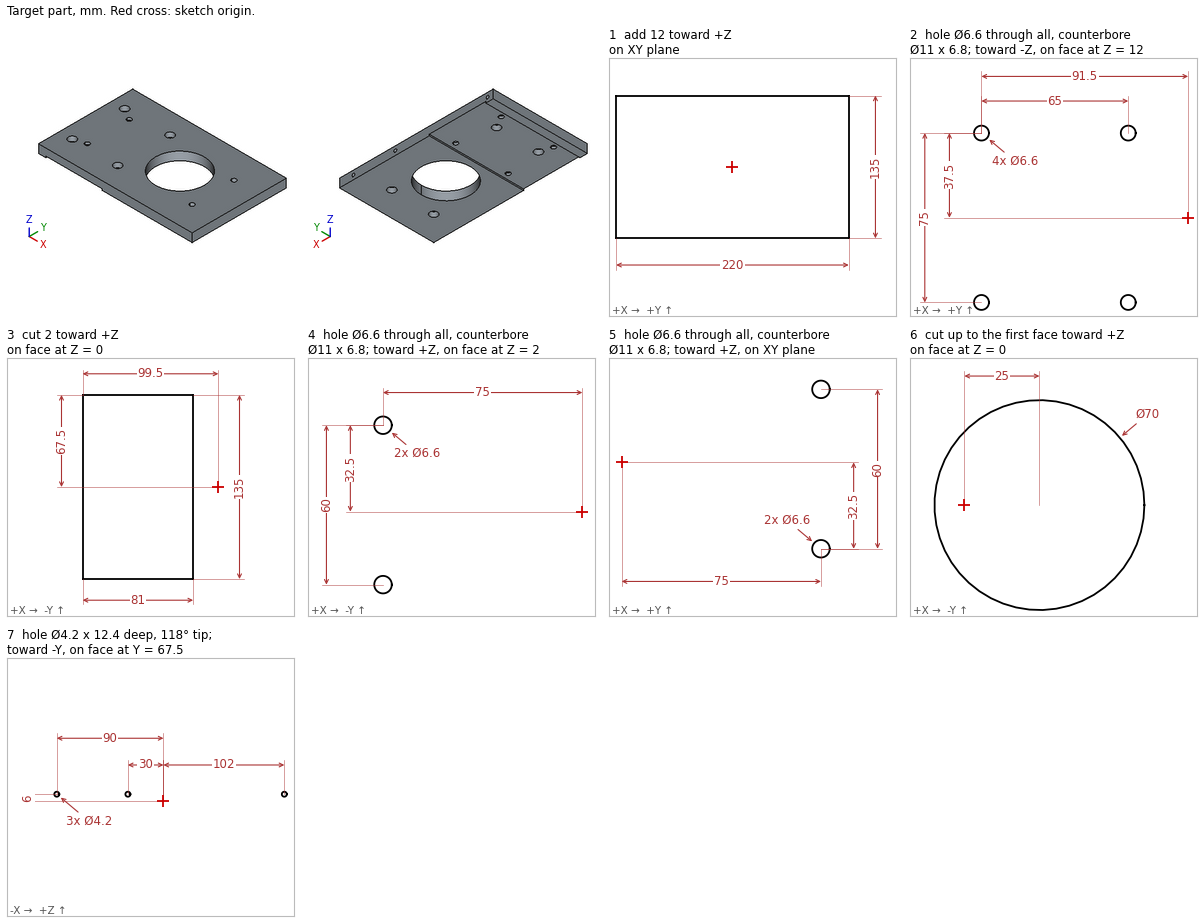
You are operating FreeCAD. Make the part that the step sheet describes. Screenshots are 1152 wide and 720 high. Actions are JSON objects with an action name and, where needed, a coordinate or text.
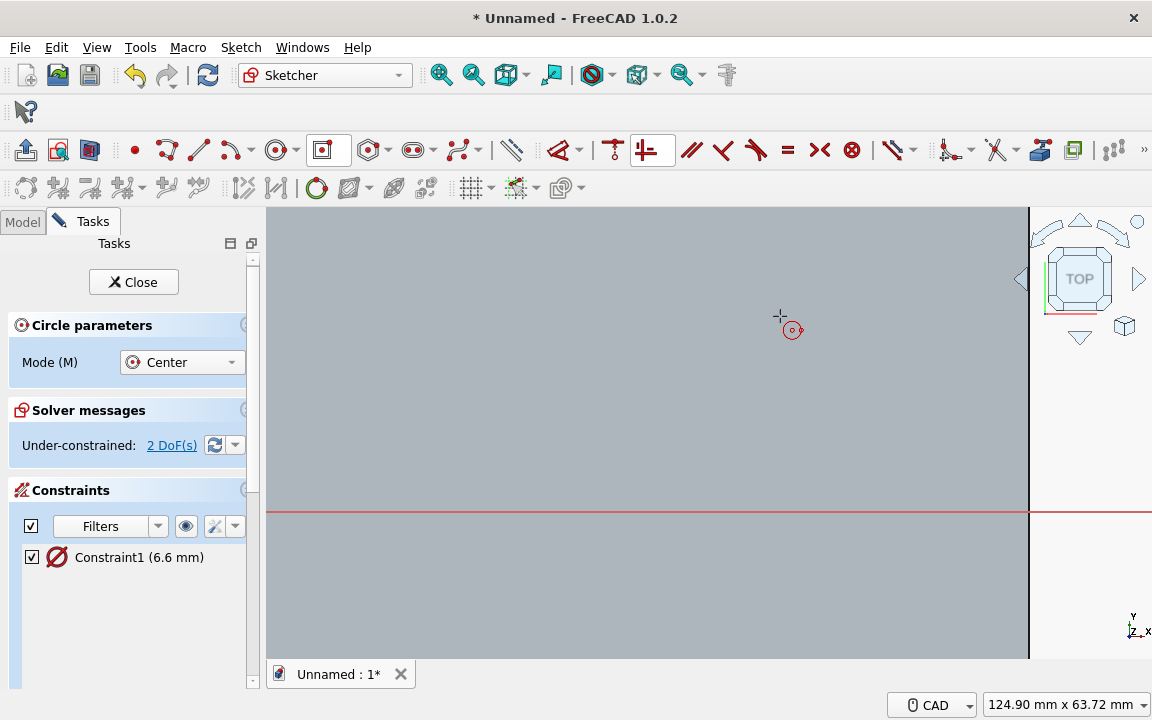
{"action": "left_click", "coordinate": [780, 317]}
{"action": "mouse_move", "coordinate": [797, 300]}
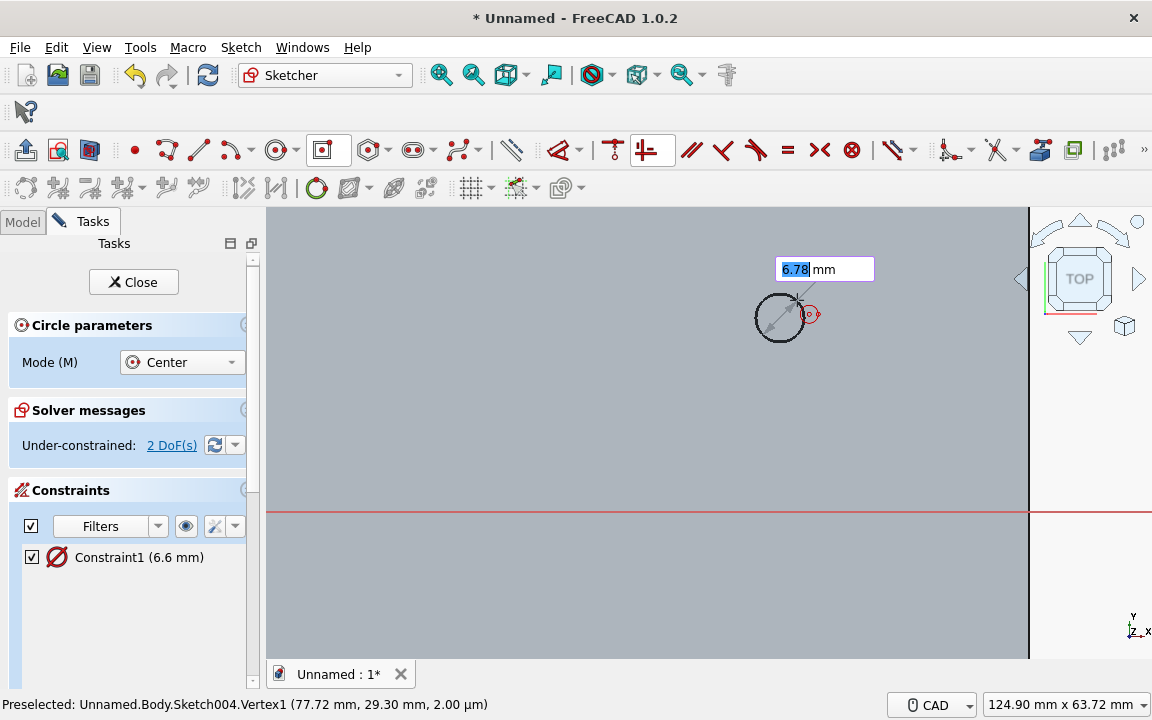
{"action": "type", "text": "6.6"}
{"action": "key", "text": "Return"}
{"action": "key", "text": "Escape"}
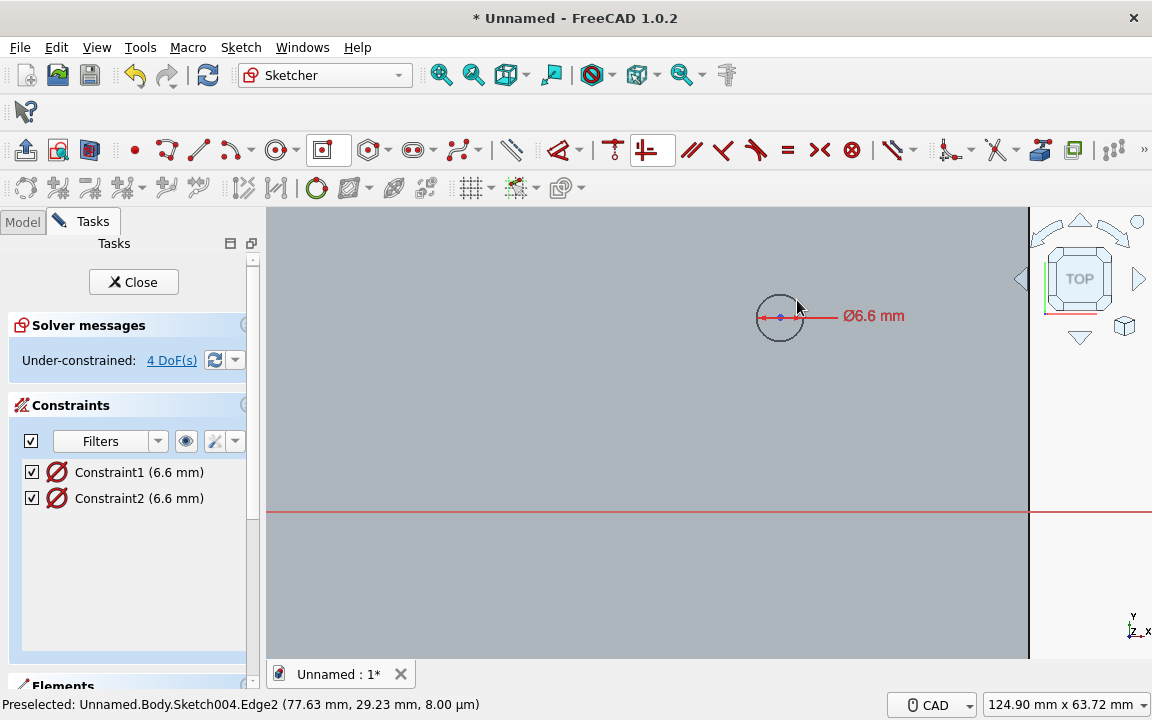
{"action": "scroll", "coordinate": [780, 316], "scroll_direction": "down", "scroll_amount": 3}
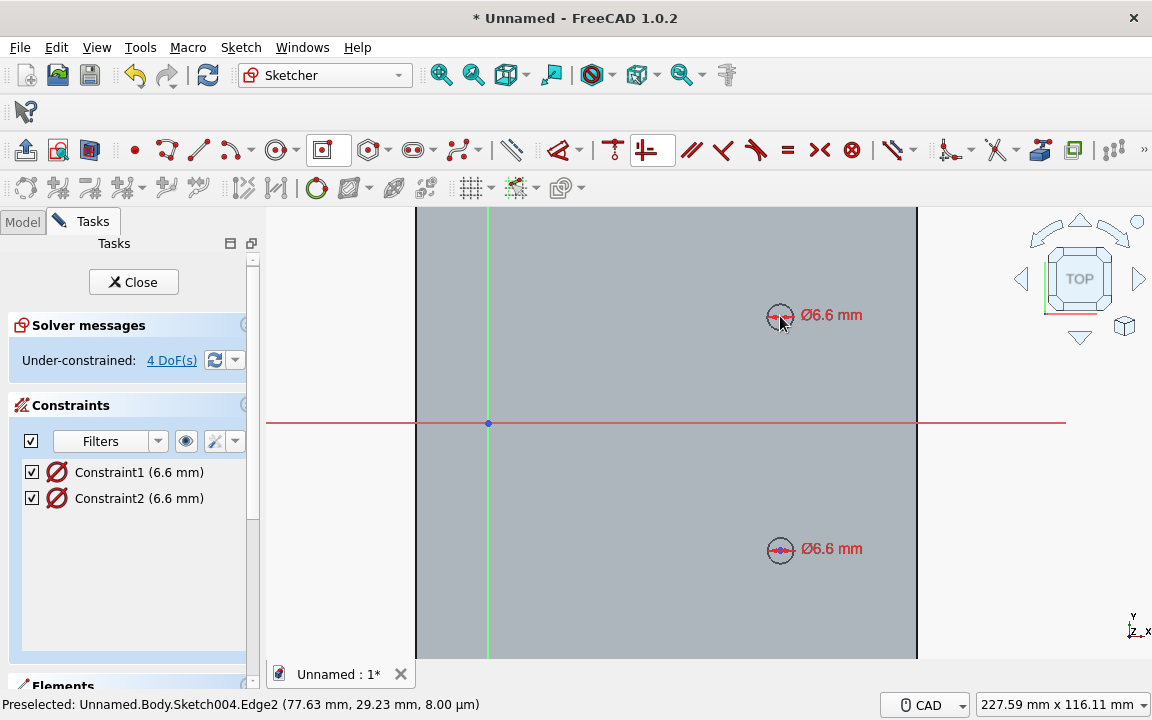
{"action": "left_click", "coordinate": [781, 551]}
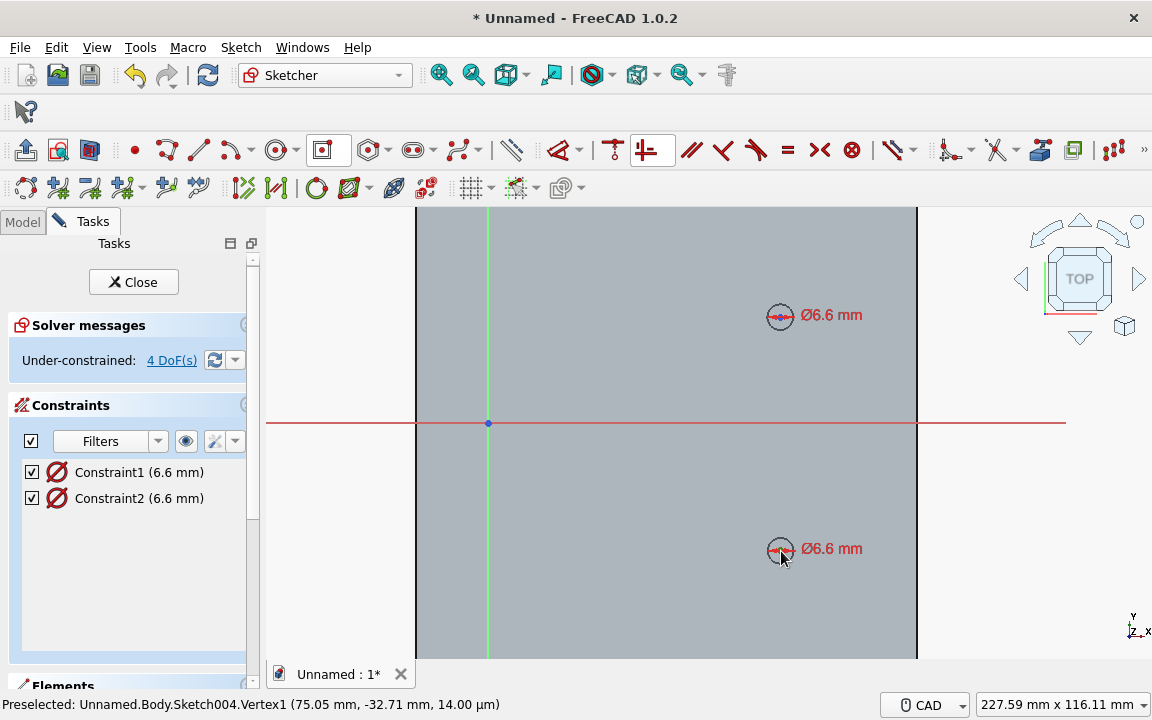
{"action": "left_click", "coordinate": [780, 317]}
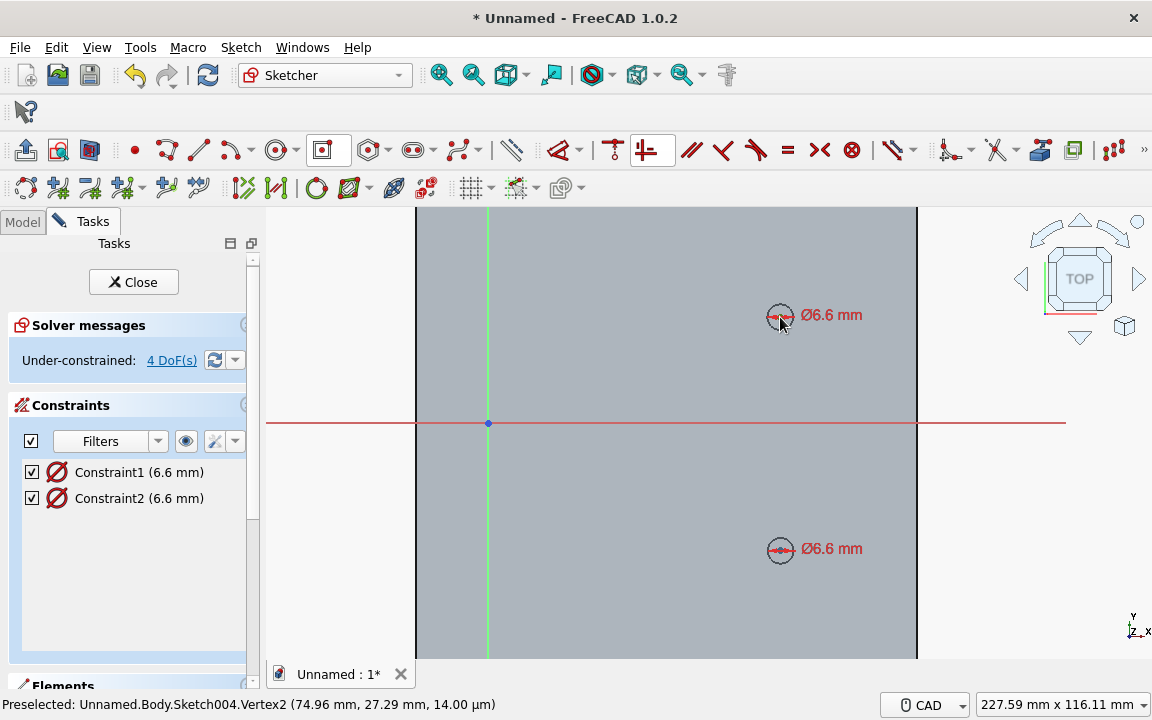
{"action": "key", "text": "v"}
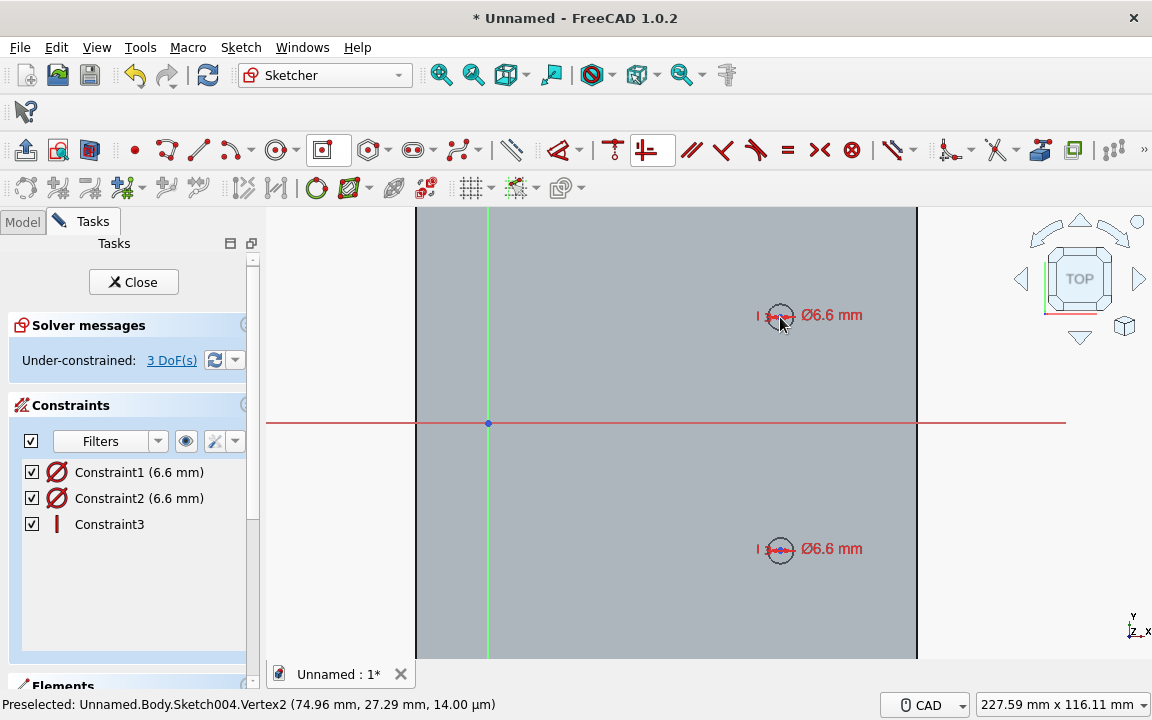
{"action": "key", "text": "d"}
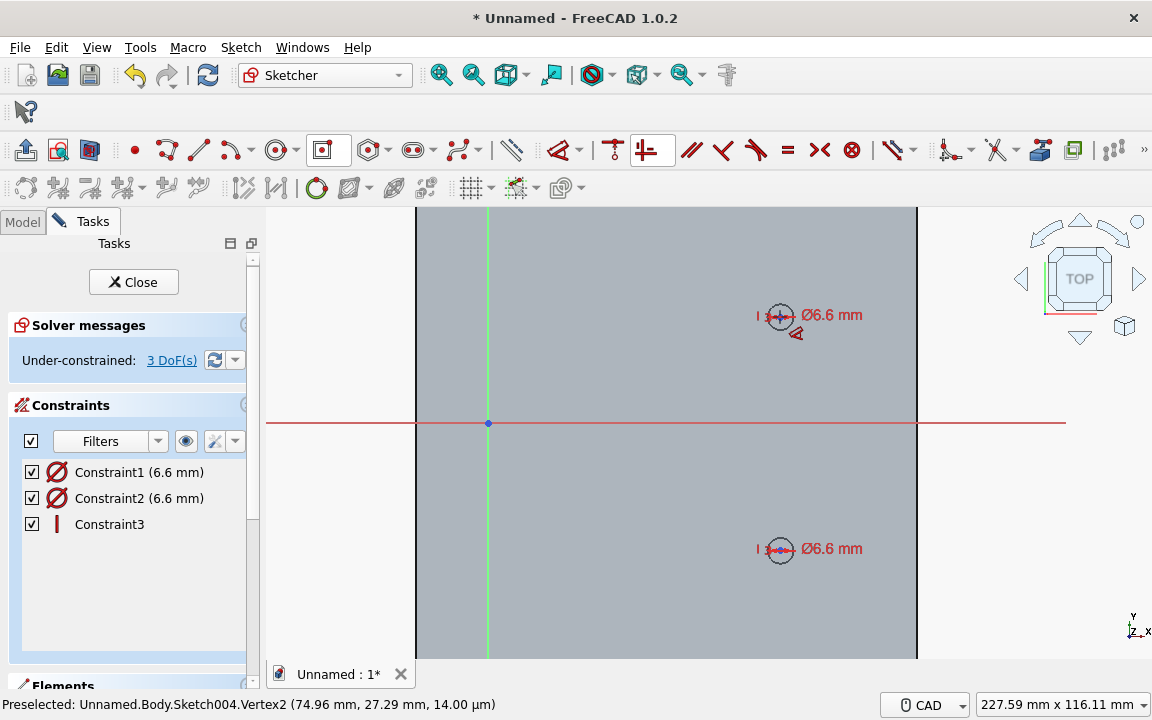
{"action": "left_click", "coordinate": [781, 551]}
{"action": "left_click", "coordinate": [635, 585]}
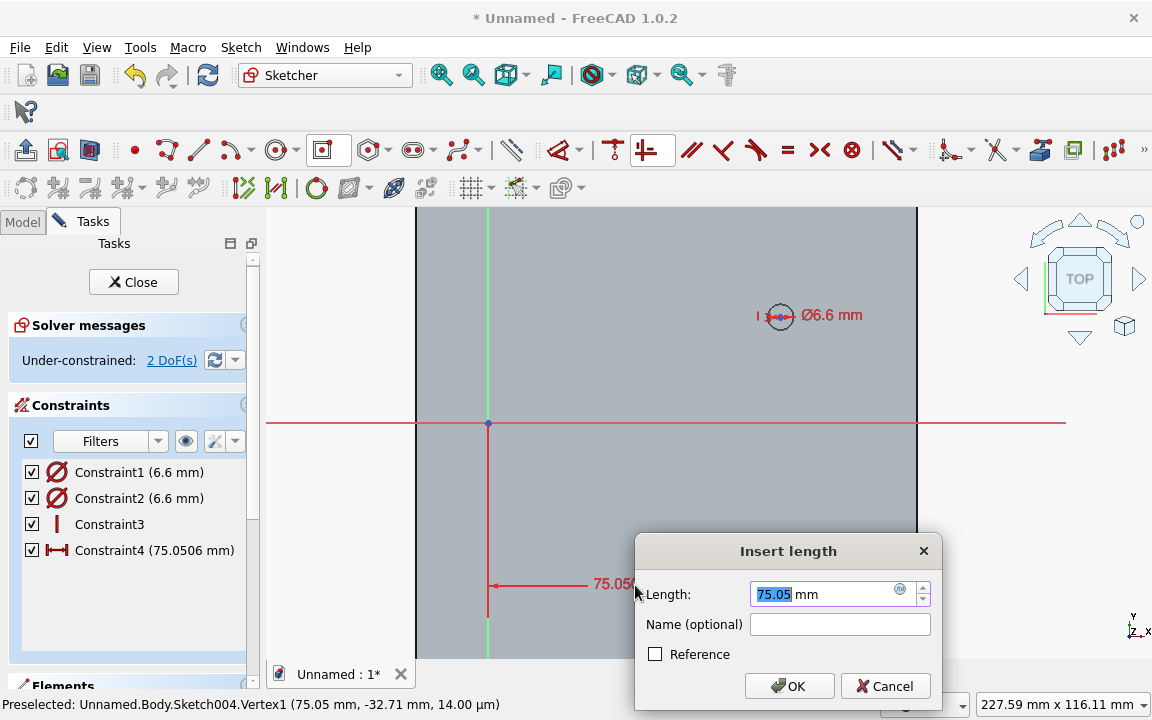
{"action": "type", "text": "75"}
{"action": "key", "text": "Return"}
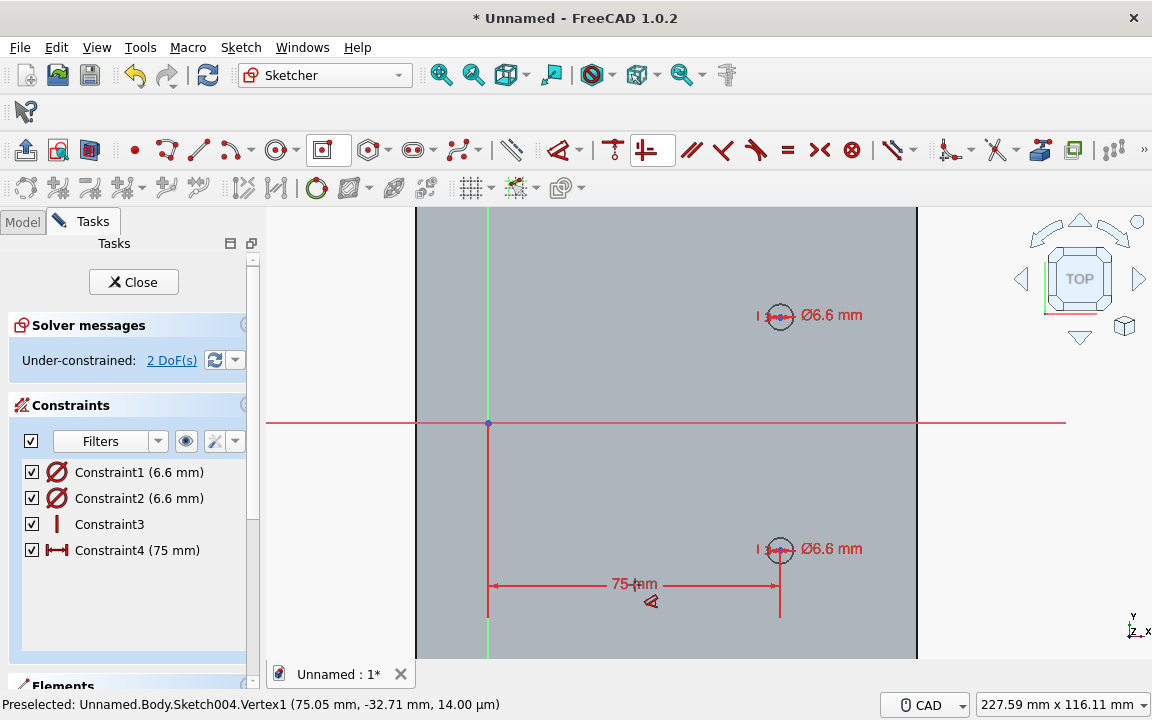
{"action": "left_click", "coordinate": [780, 551]}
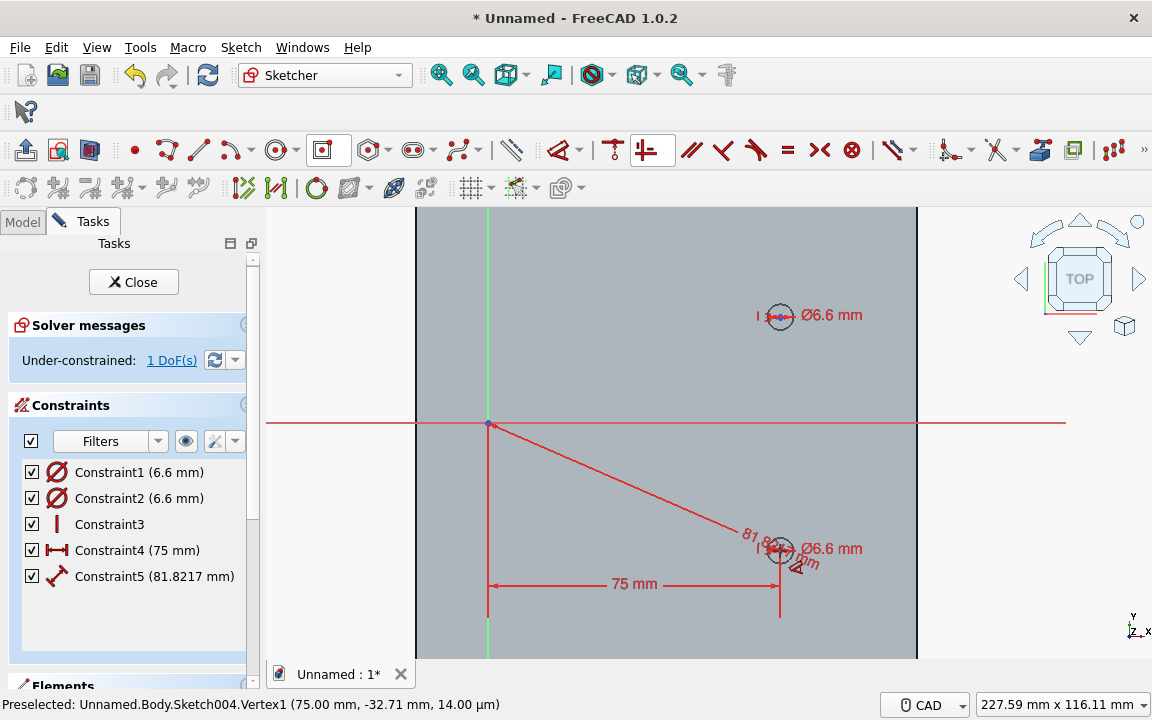
{"action": "left_click", "coordinate": [780, 317]}
{"action": "left_click", "coordinate": [814, 380]}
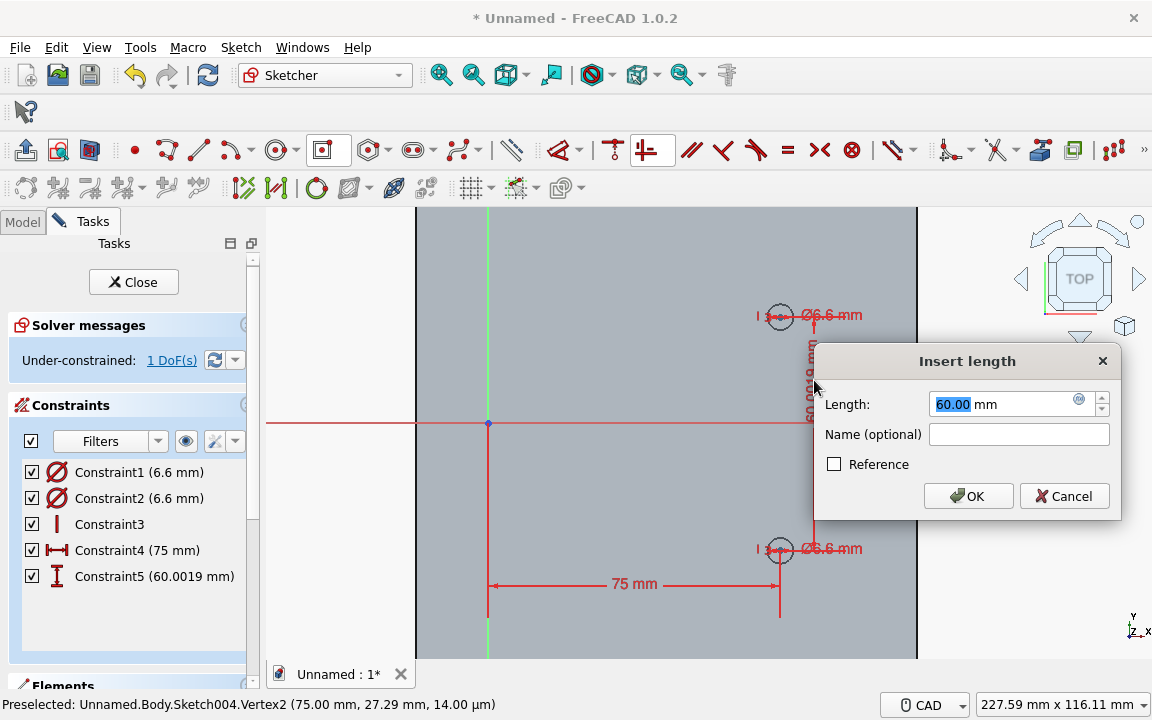
{"action": "type", "text": "60"}
{"action": "key", "text": "Return"}